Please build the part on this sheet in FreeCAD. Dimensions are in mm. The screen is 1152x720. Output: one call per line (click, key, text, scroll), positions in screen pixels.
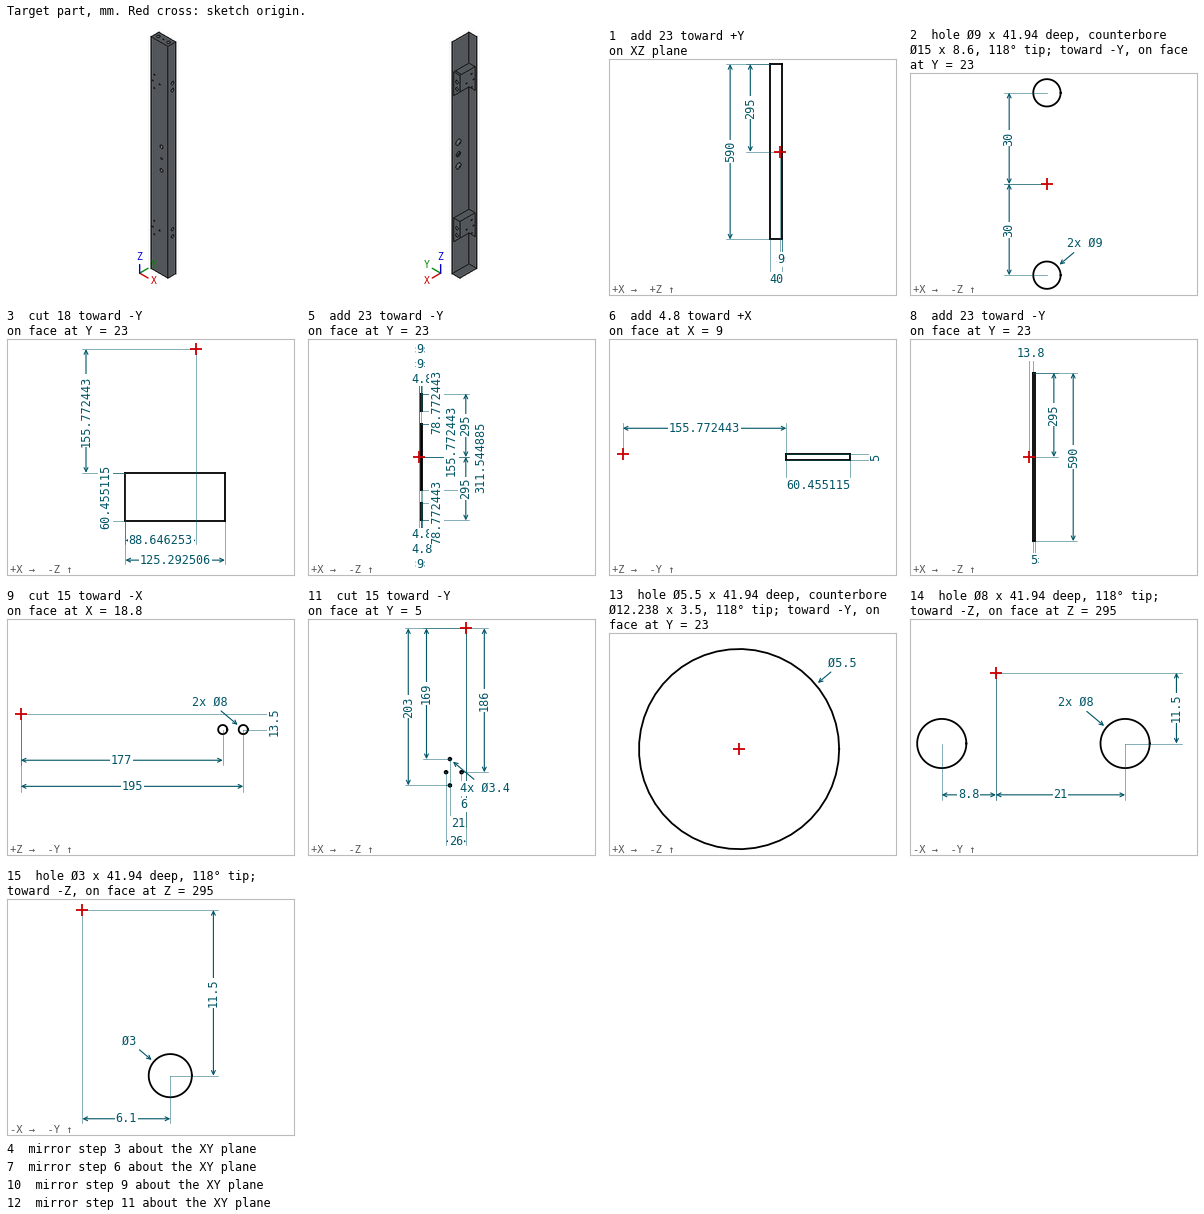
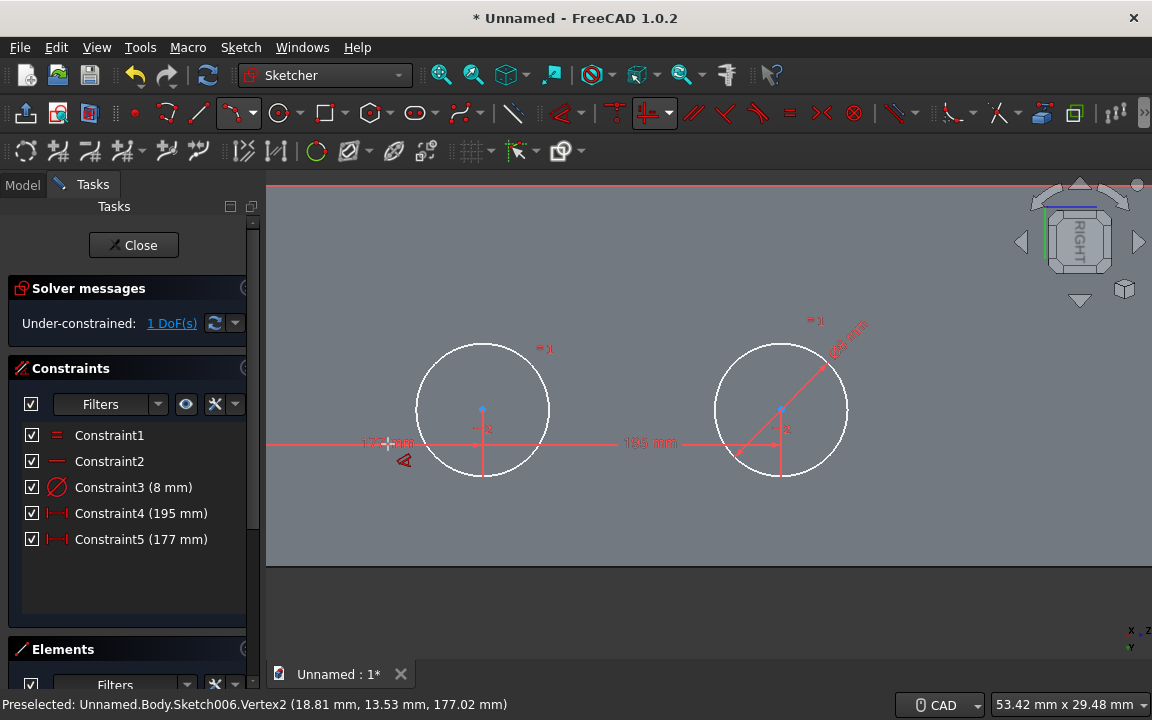
click(781, 410)
click(815, 304)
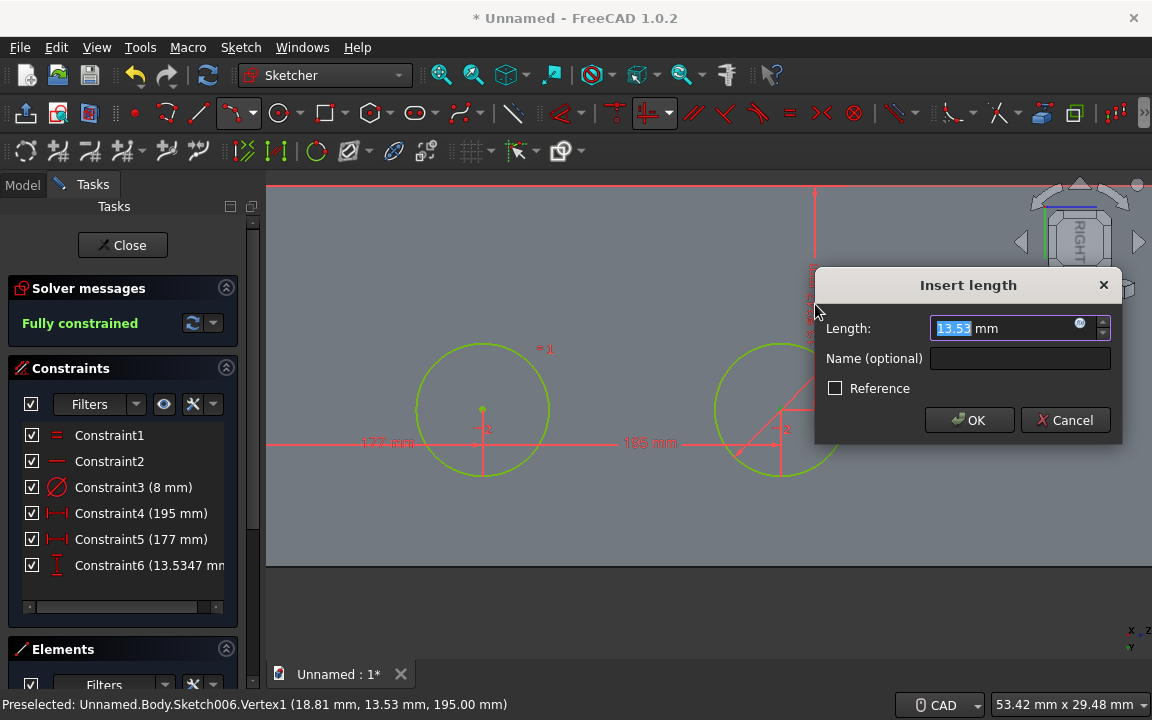
text(13.5)
key(Return)
key(Escape)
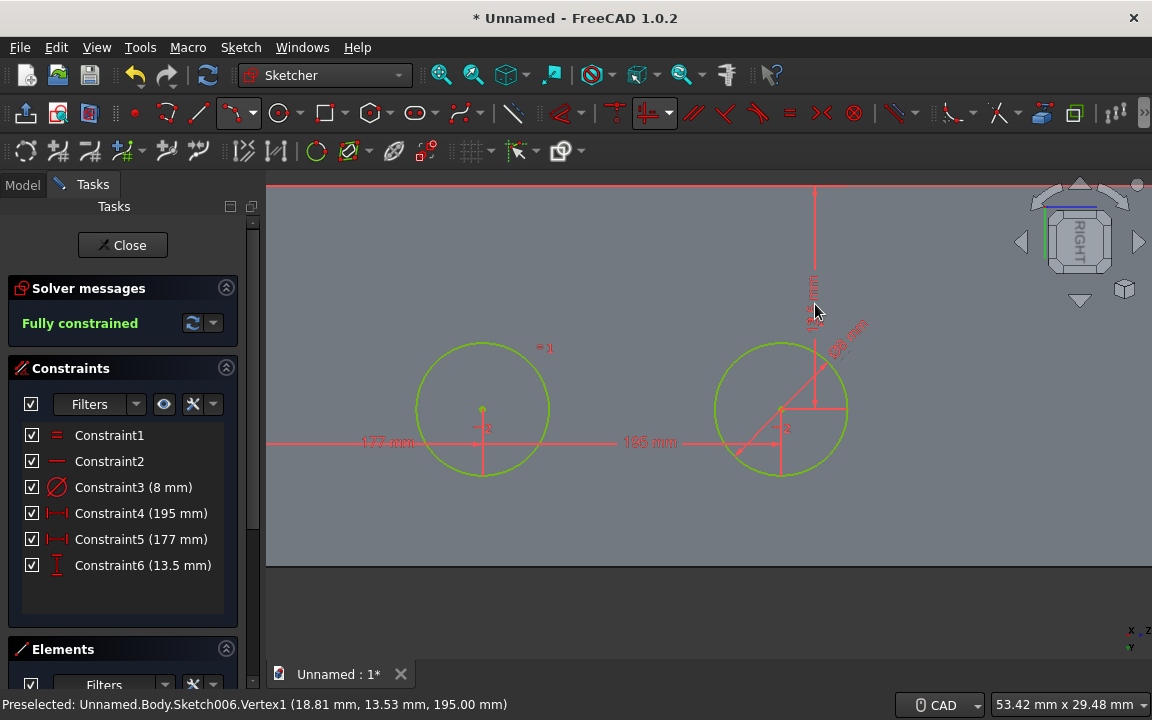
click(123, 245)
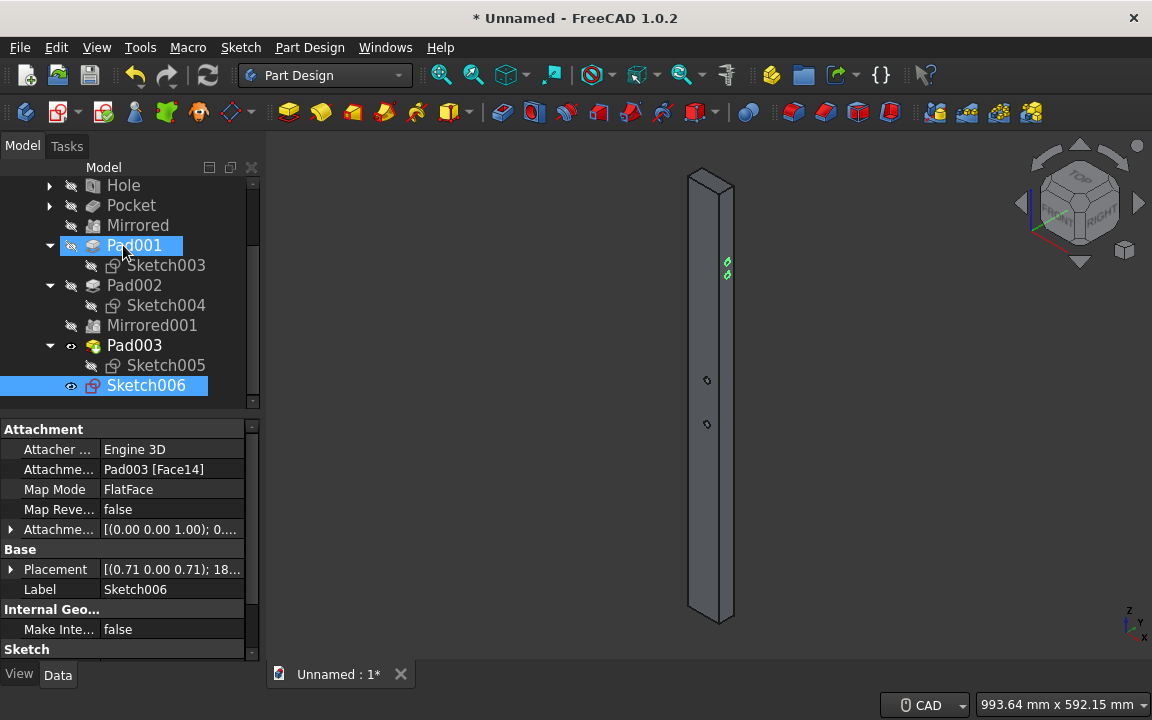
click(504, 112)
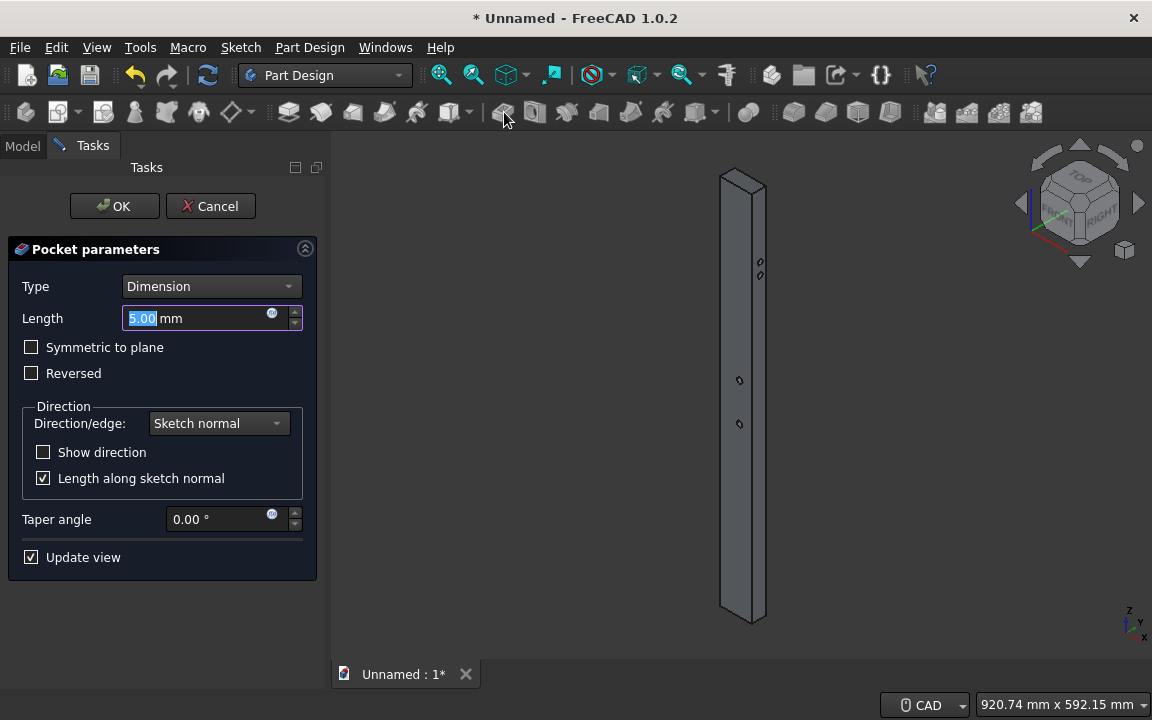
text(15)
key(Tab)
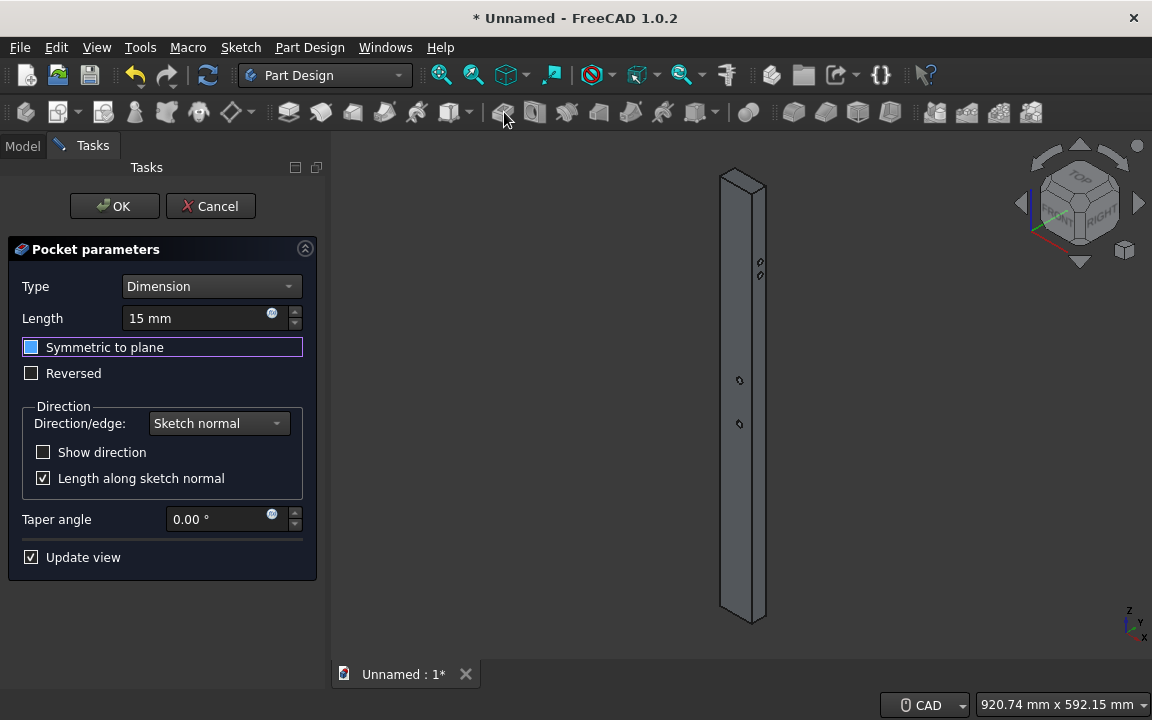
click(115, 206)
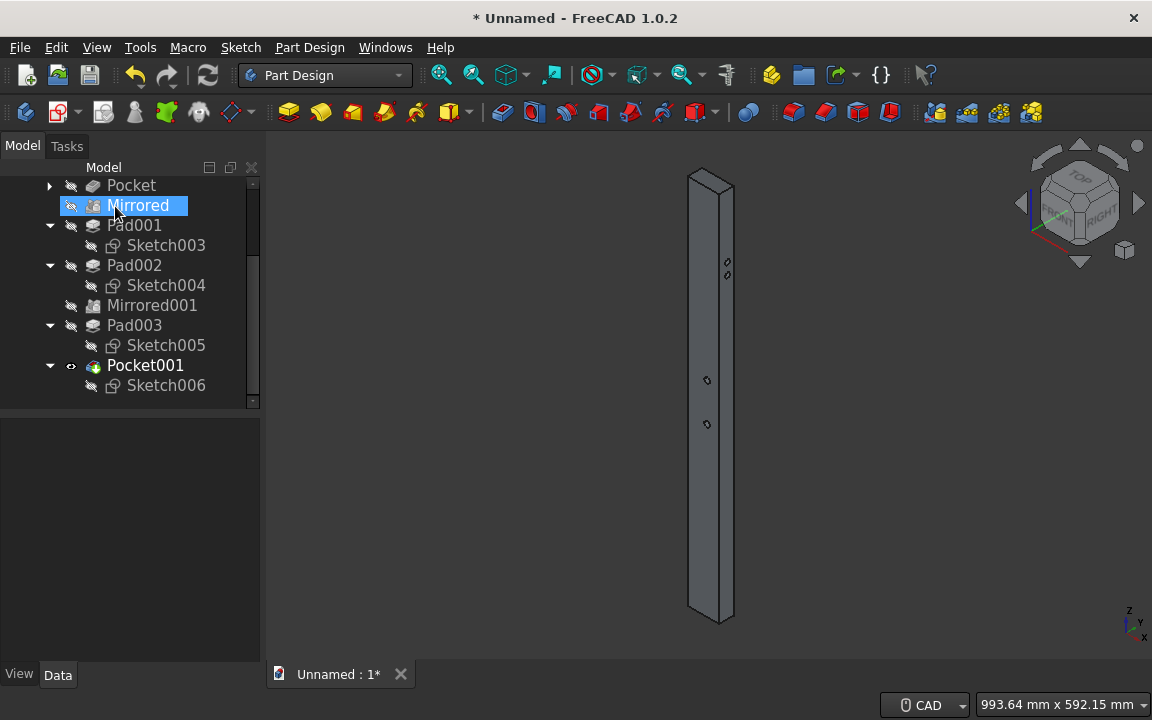
click(116, 366)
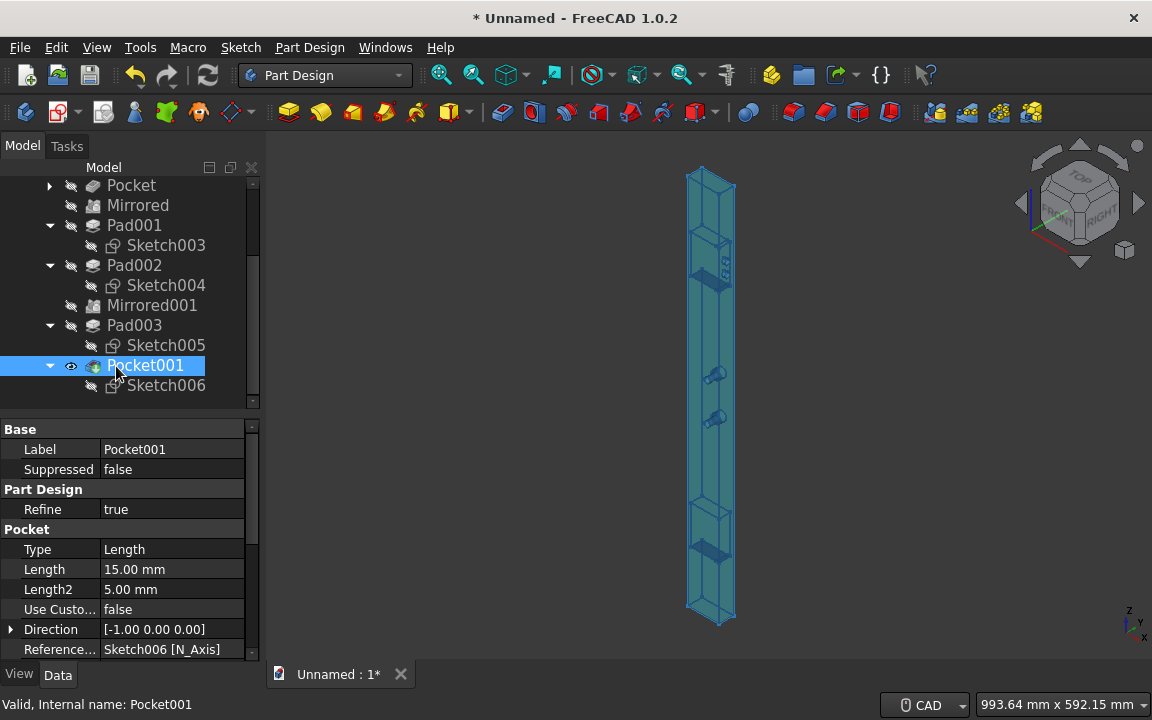
click(936, 112)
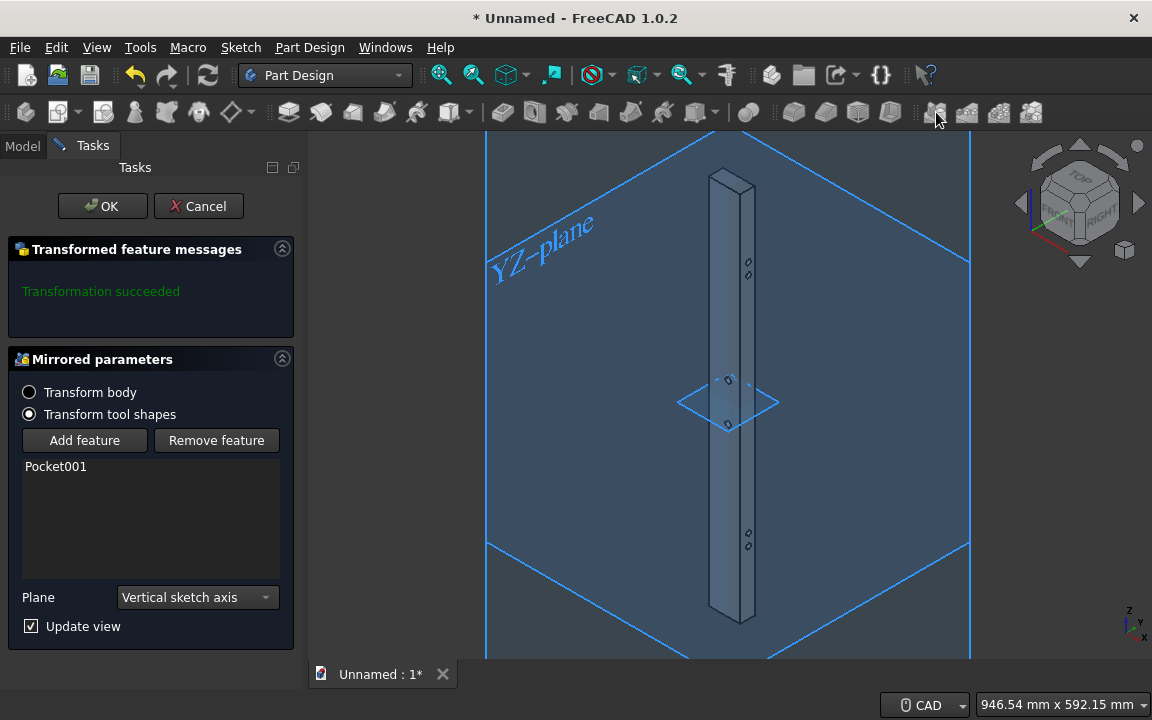
click(198, 598)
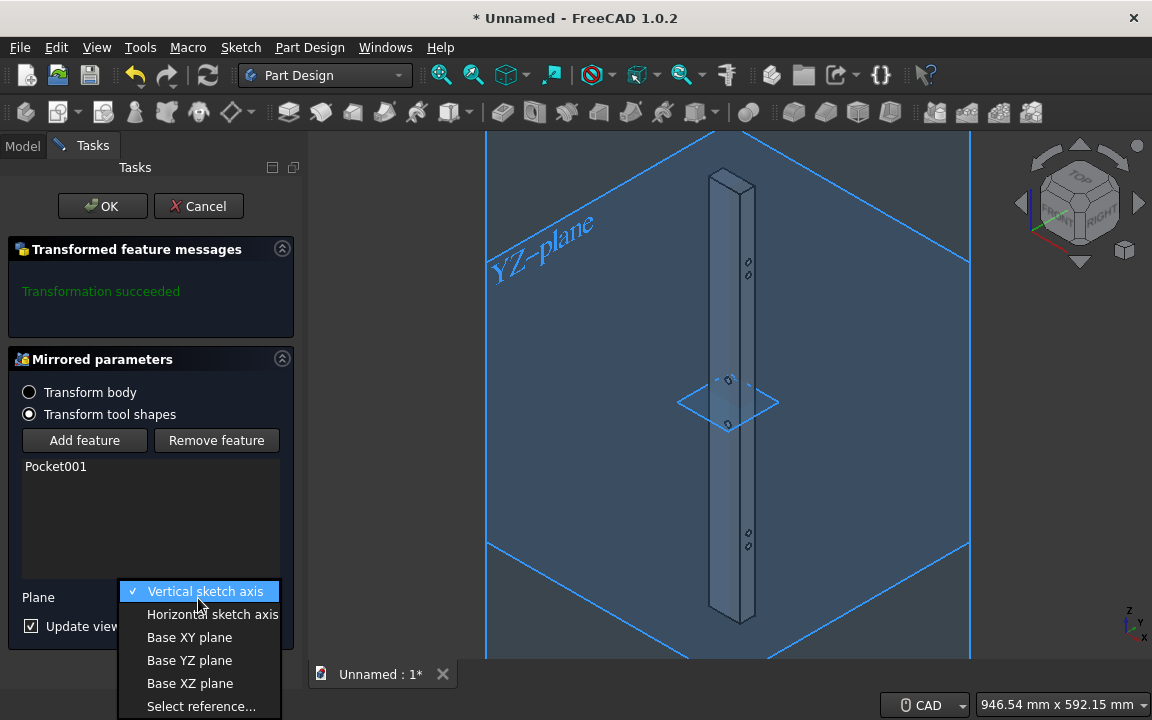
click(198, 638)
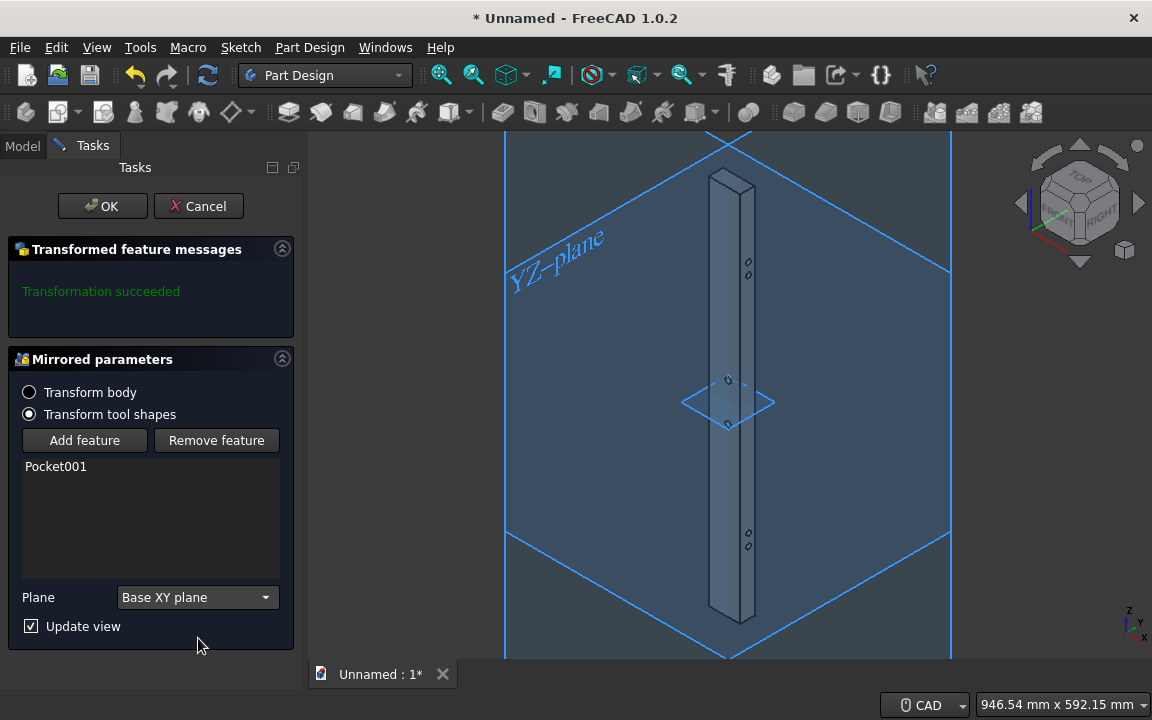
click(103, 206)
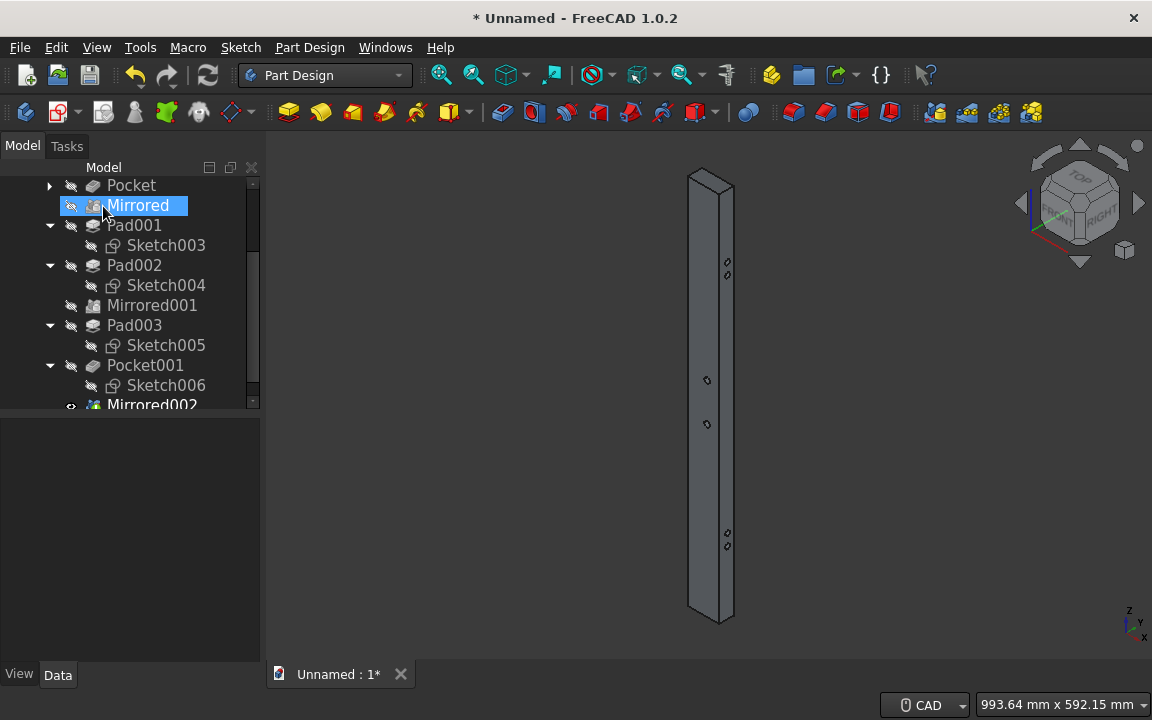
key(4)